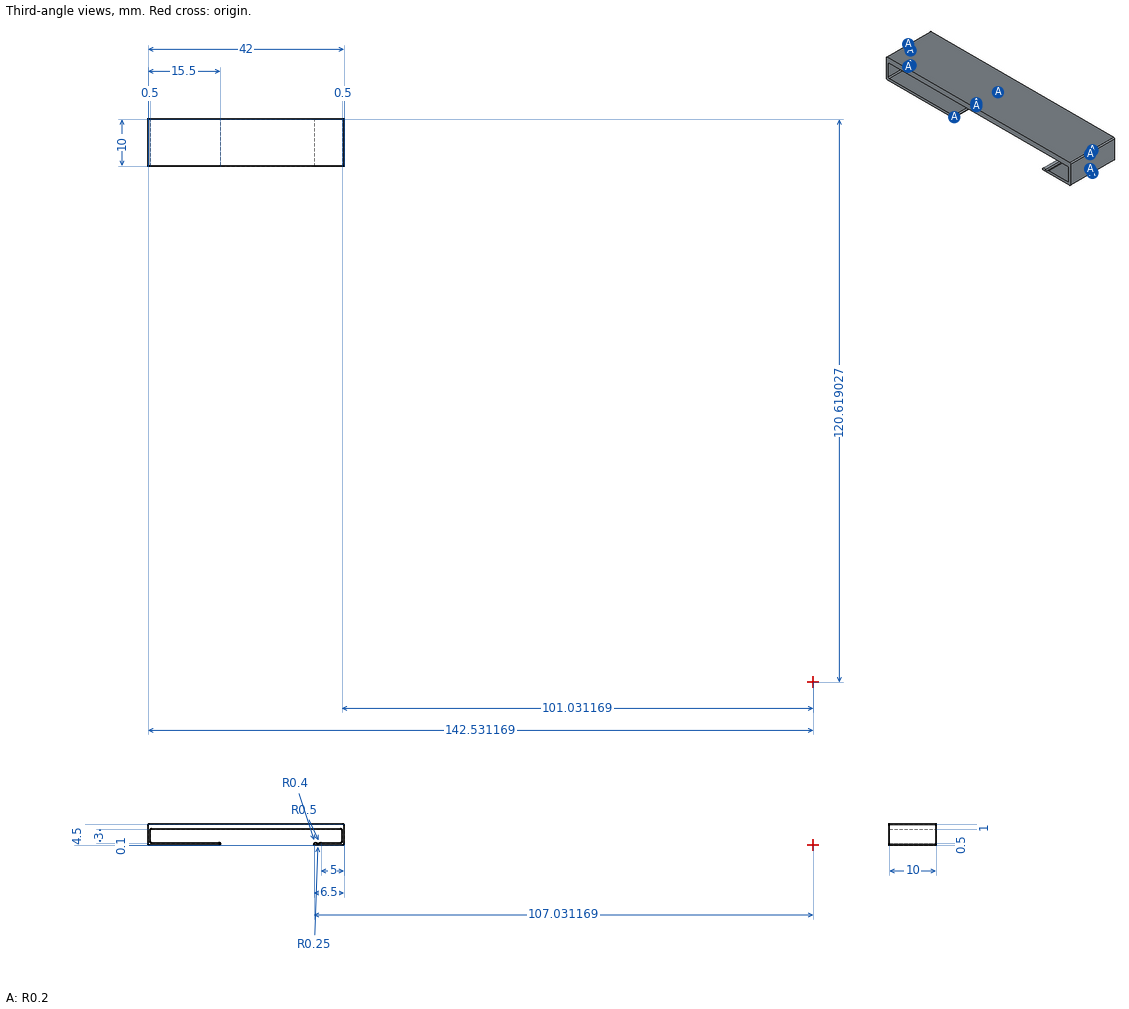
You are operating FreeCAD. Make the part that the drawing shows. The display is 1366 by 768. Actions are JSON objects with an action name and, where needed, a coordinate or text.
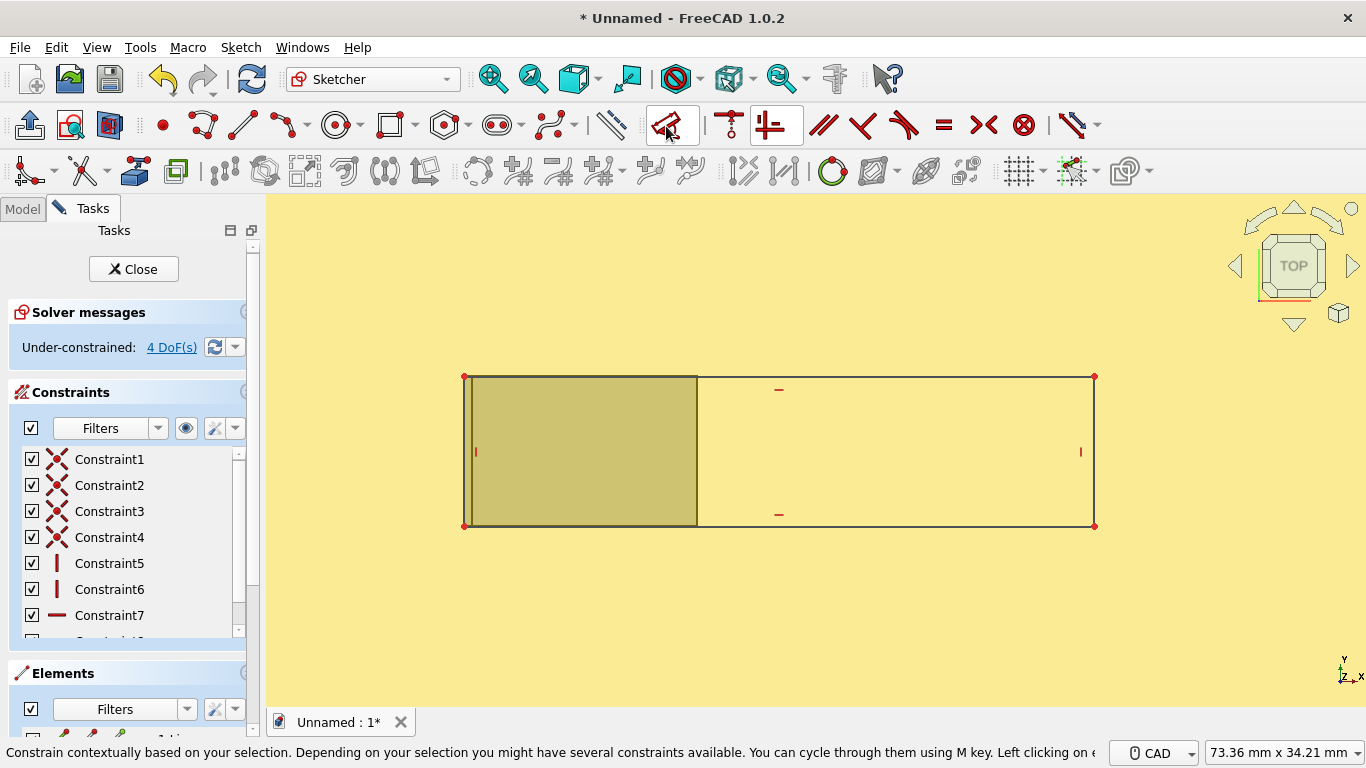
{"action": "left_click", "coordinate": [464, 422]}
{"action": "left_click", "coordinate": [430, 452]}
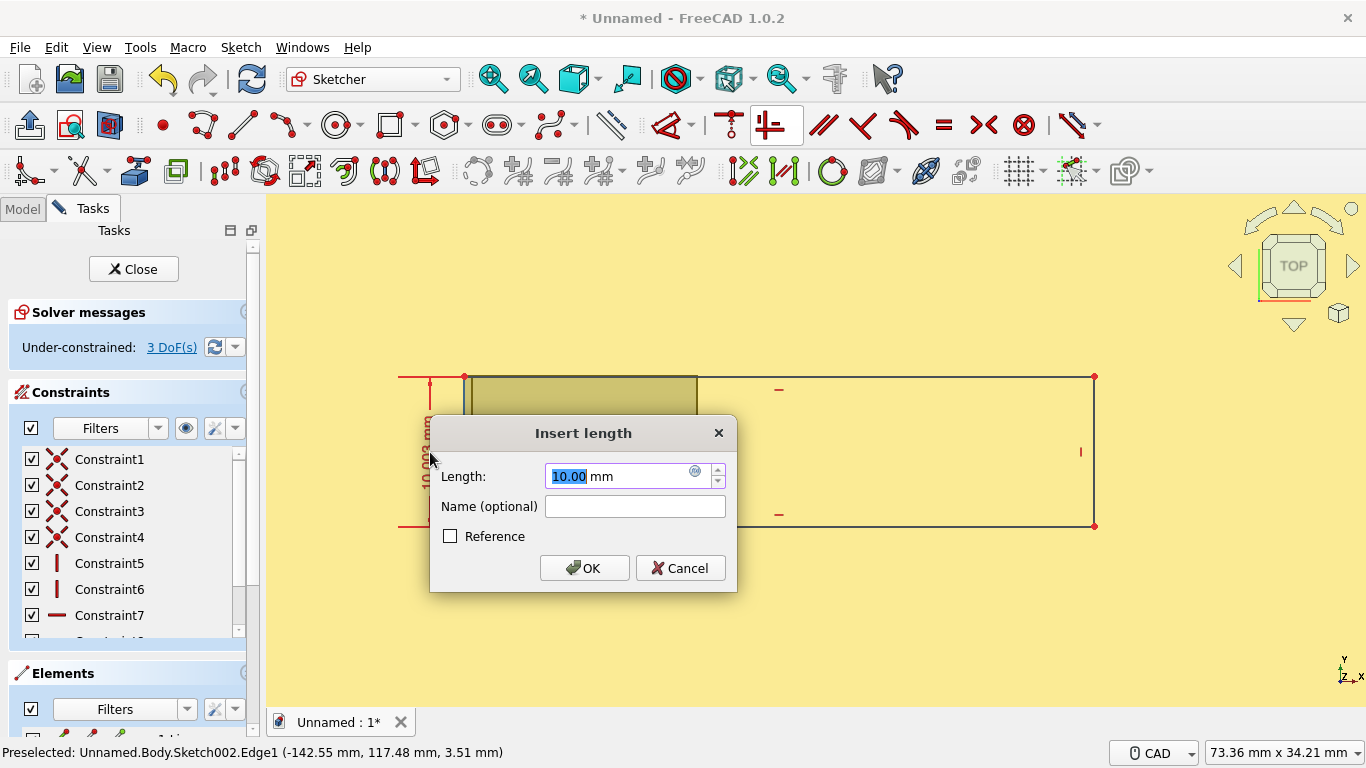
{"action": "type", "text": "10"}
{"action": "key", "text": "Return"}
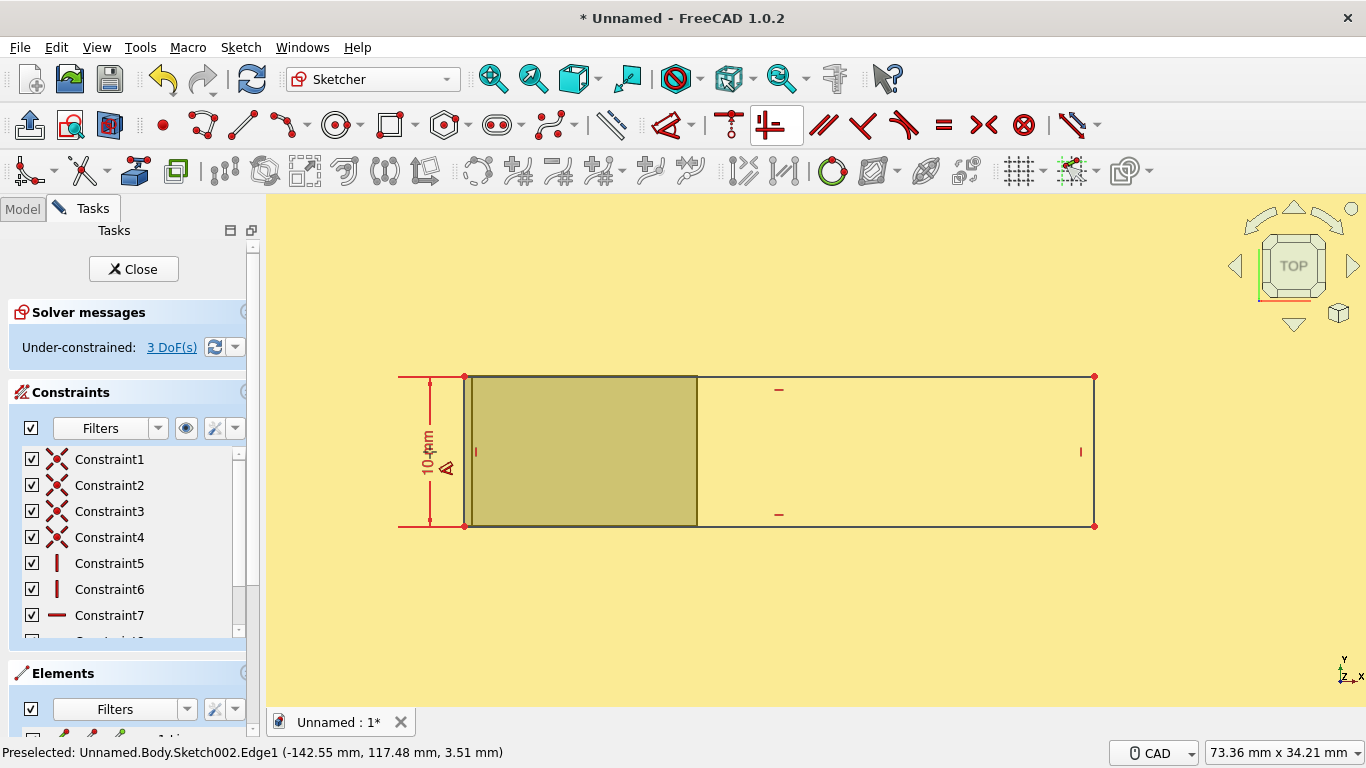
{"action": "left_click", "coordinate": [653, 527]}
{"action": "left_click", "coordinate": [779, 561]}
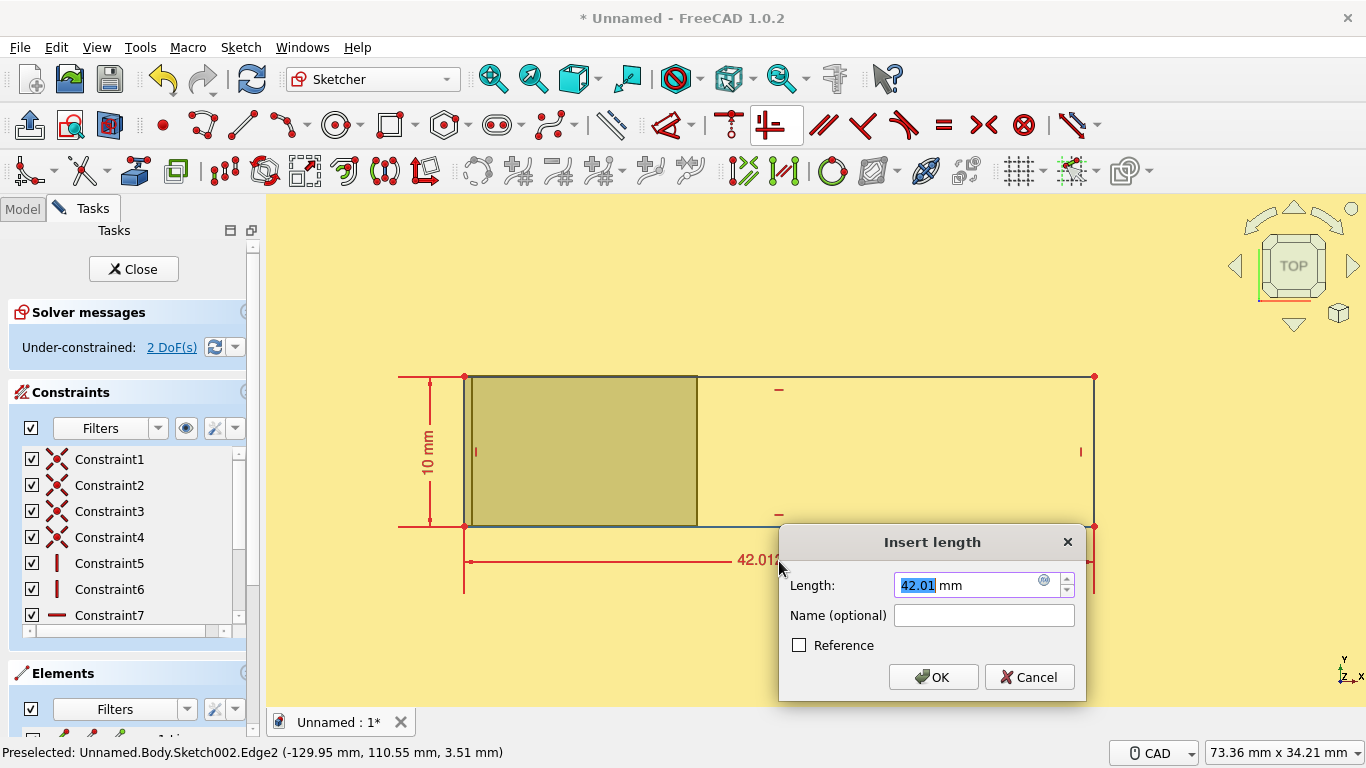
{"action": "type", "text": "42"}
{"action": "key", "text": "Return"}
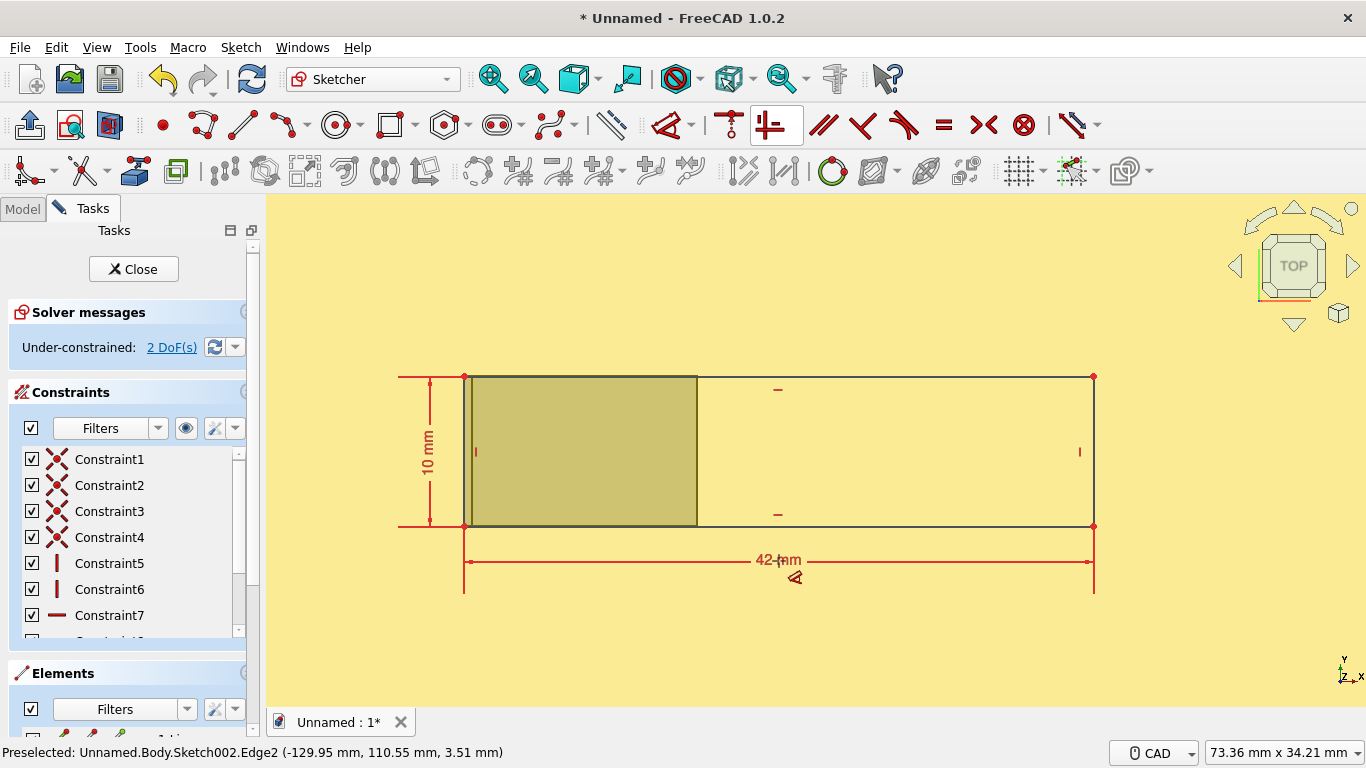
{"action": "left_click", "coordinate": [464, 377]}
{"action": "left_click", "coordinate": [832, 343]}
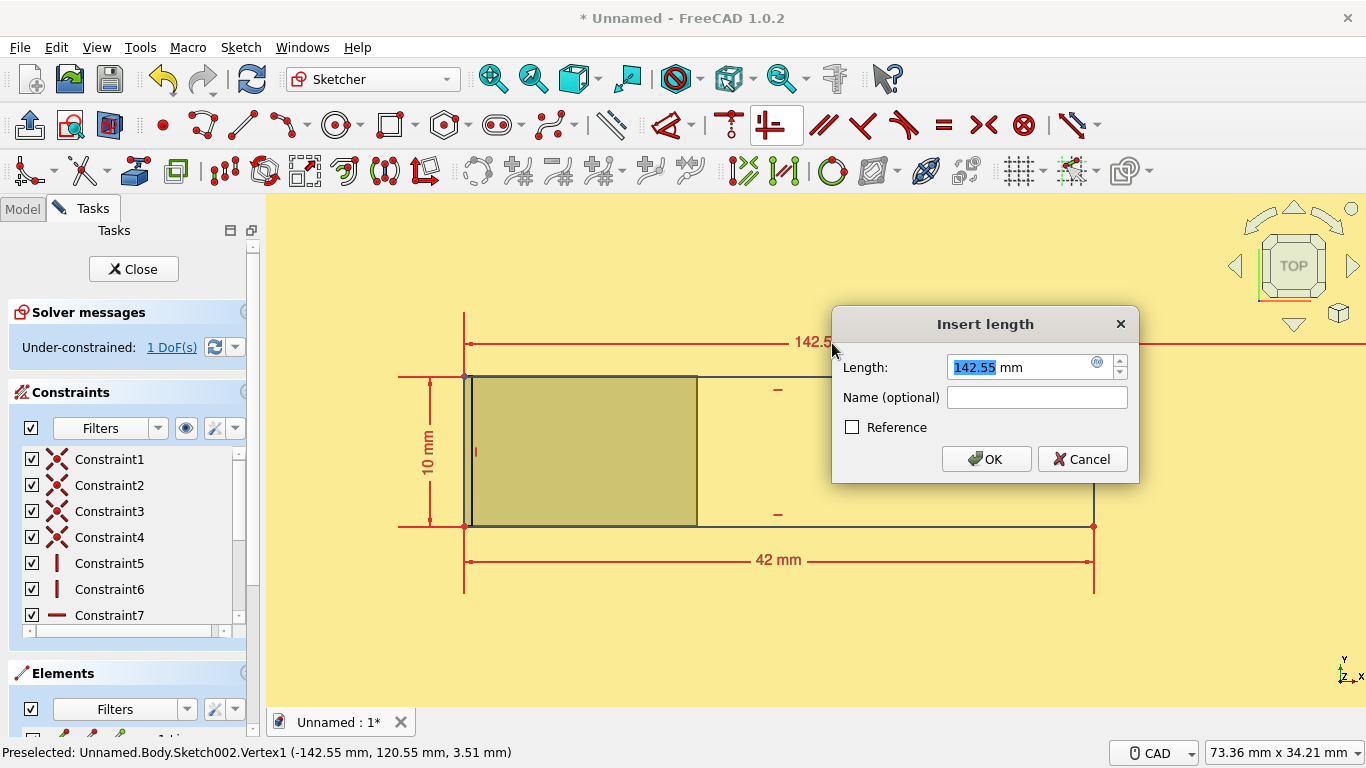
{"action": "type", "text": "142.531169"}
{"action": "key", "text": "Return"}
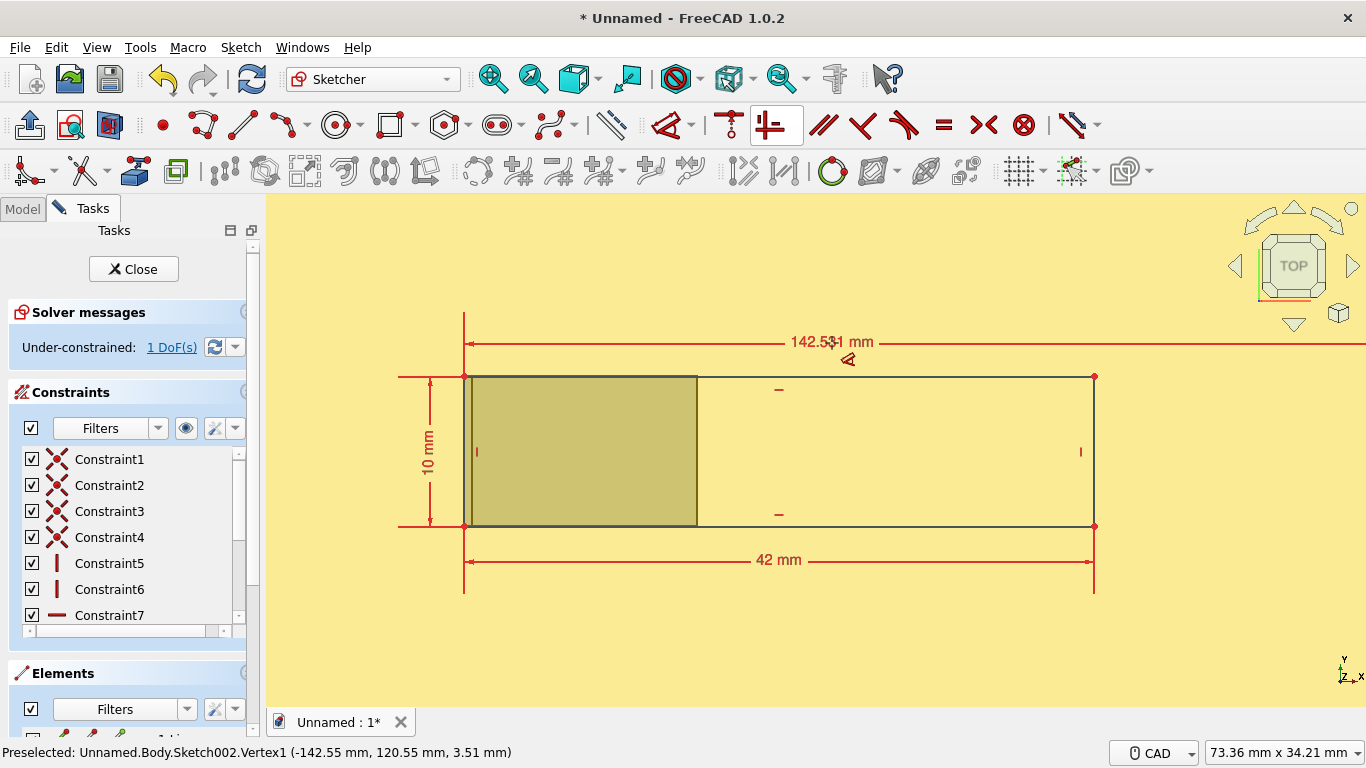
{"action": "left_click", "coordinate": [464, 377]}
{"action": "left_click", "coordinate": [430, 528]}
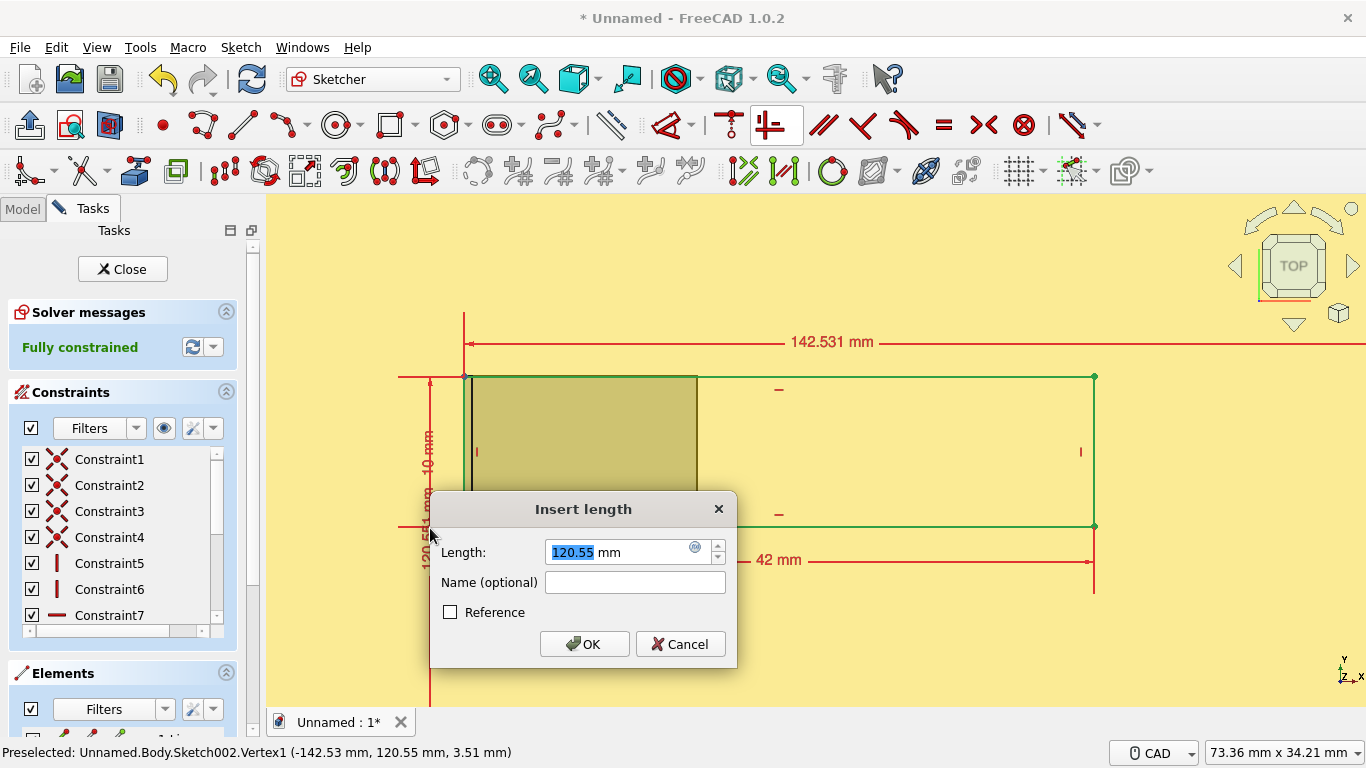
{"action": "type", "text": "120.619027"}
{"action": "key", "text": "Return"}
{"action": "key", "text": "Escape"}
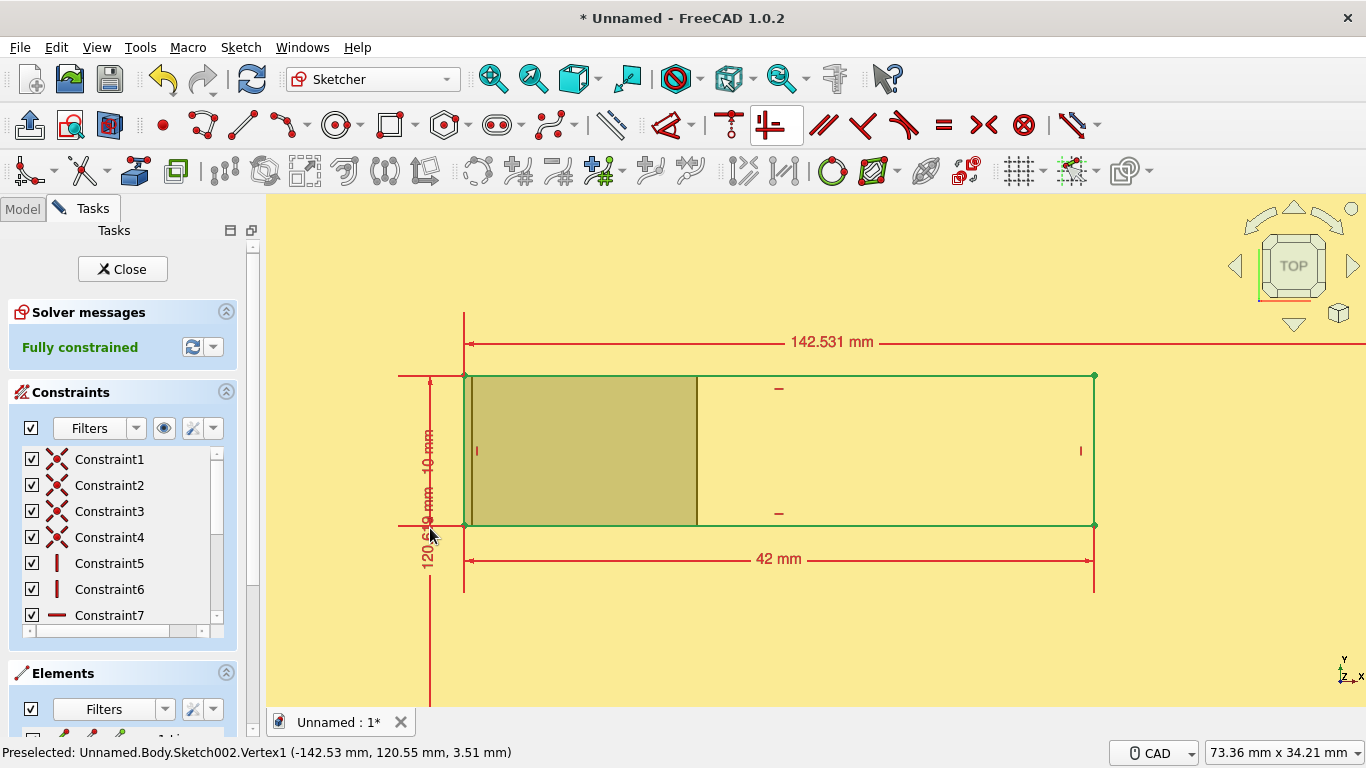
{"action": "left_click", "coordinate": [123, 269]}